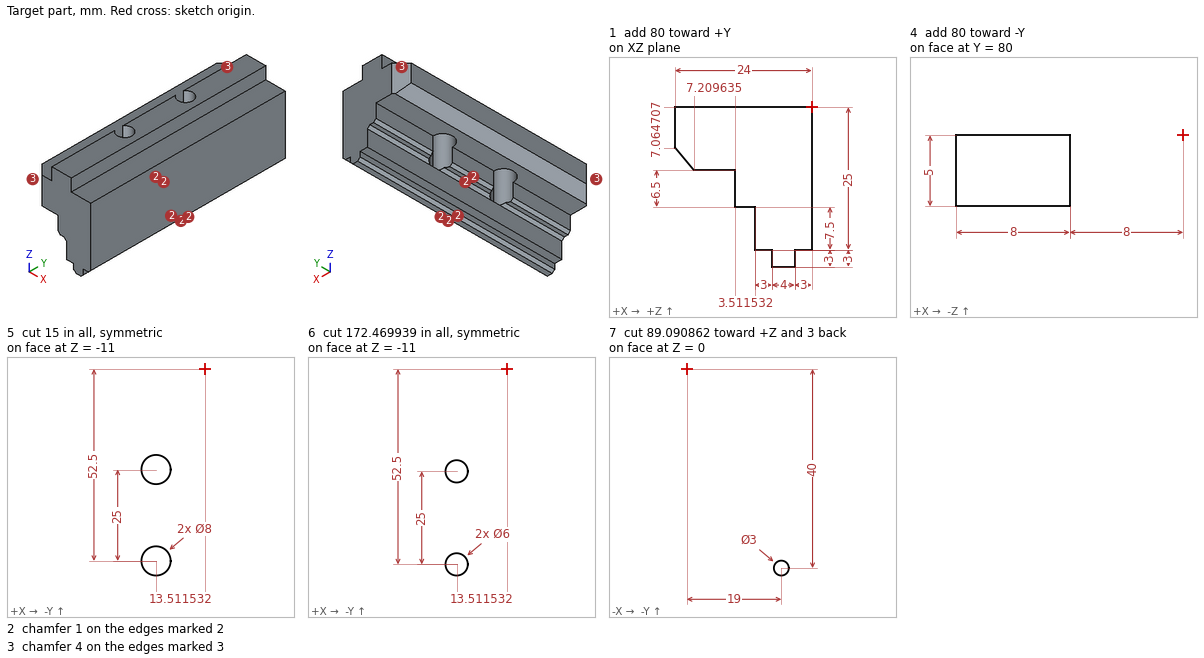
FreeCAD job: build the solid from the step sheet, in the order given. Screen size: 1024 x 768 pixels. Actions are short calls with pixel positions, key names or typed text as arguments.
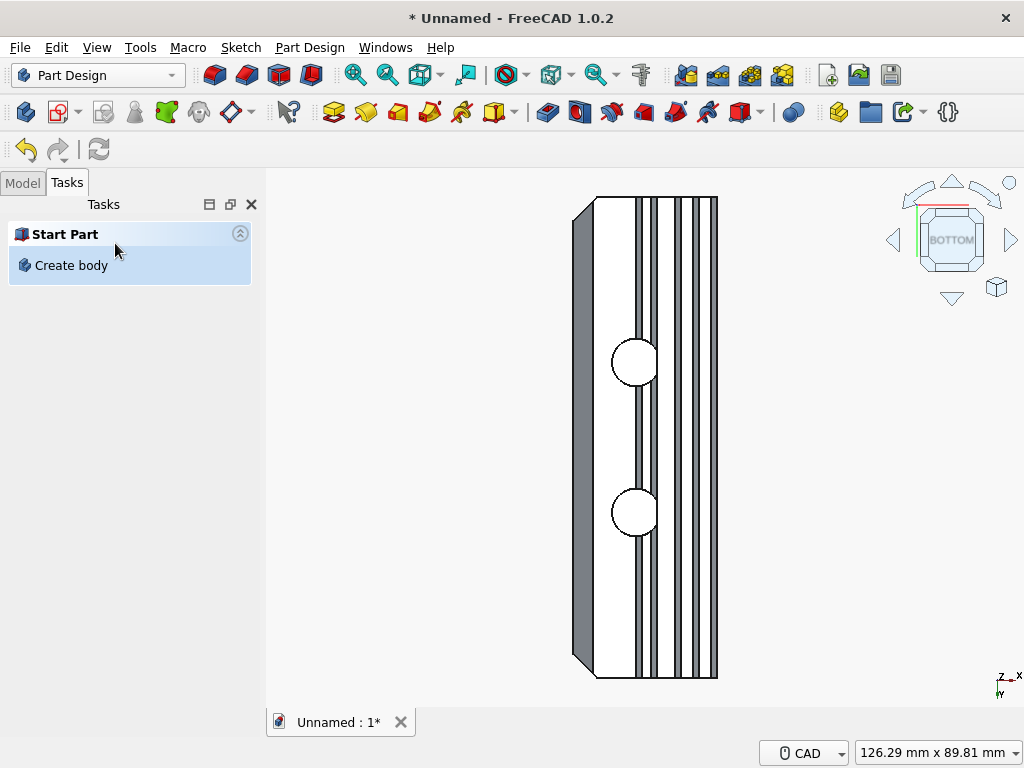
click(614, 642)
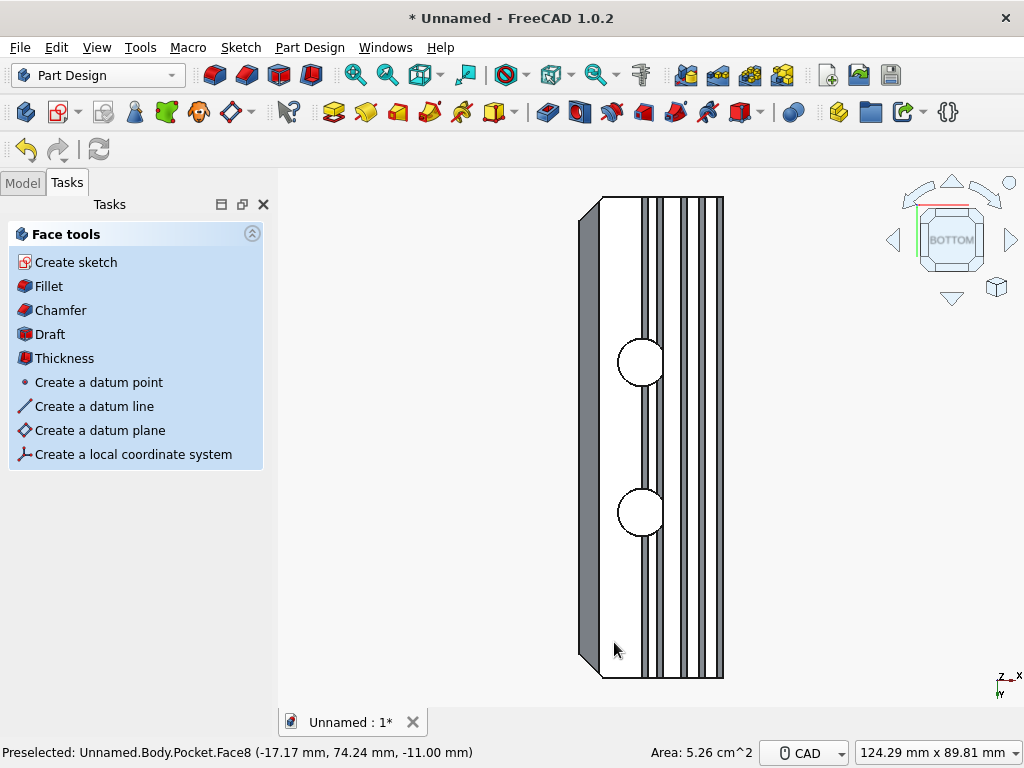
click(58, 112)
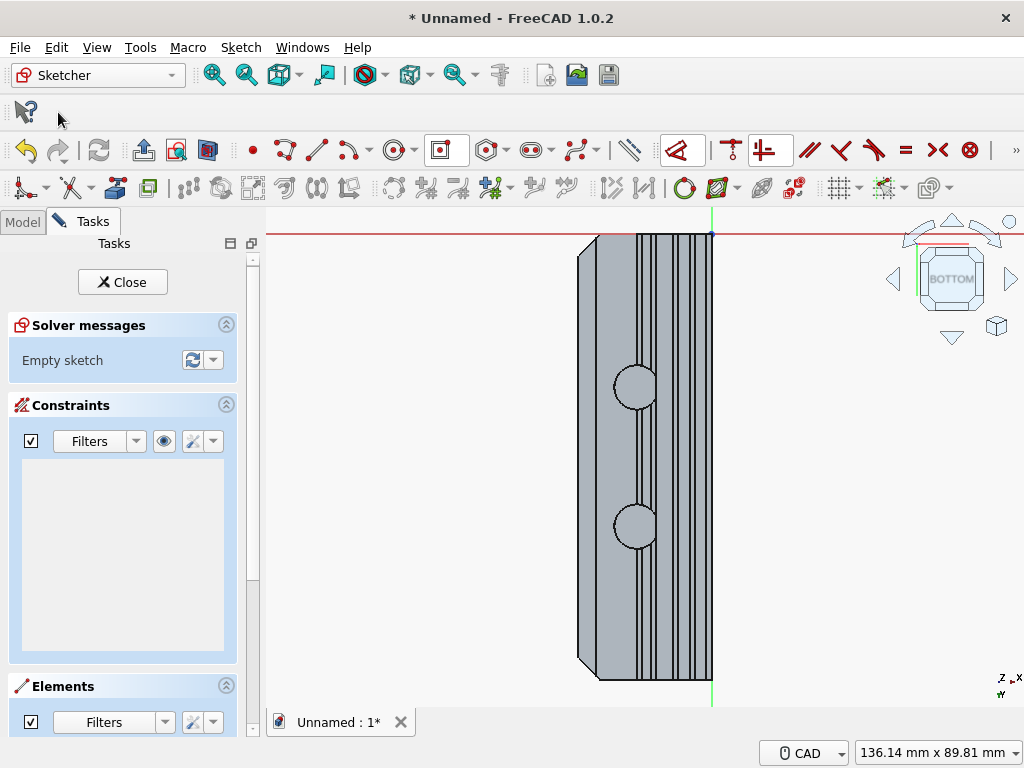
key(q)
key(s)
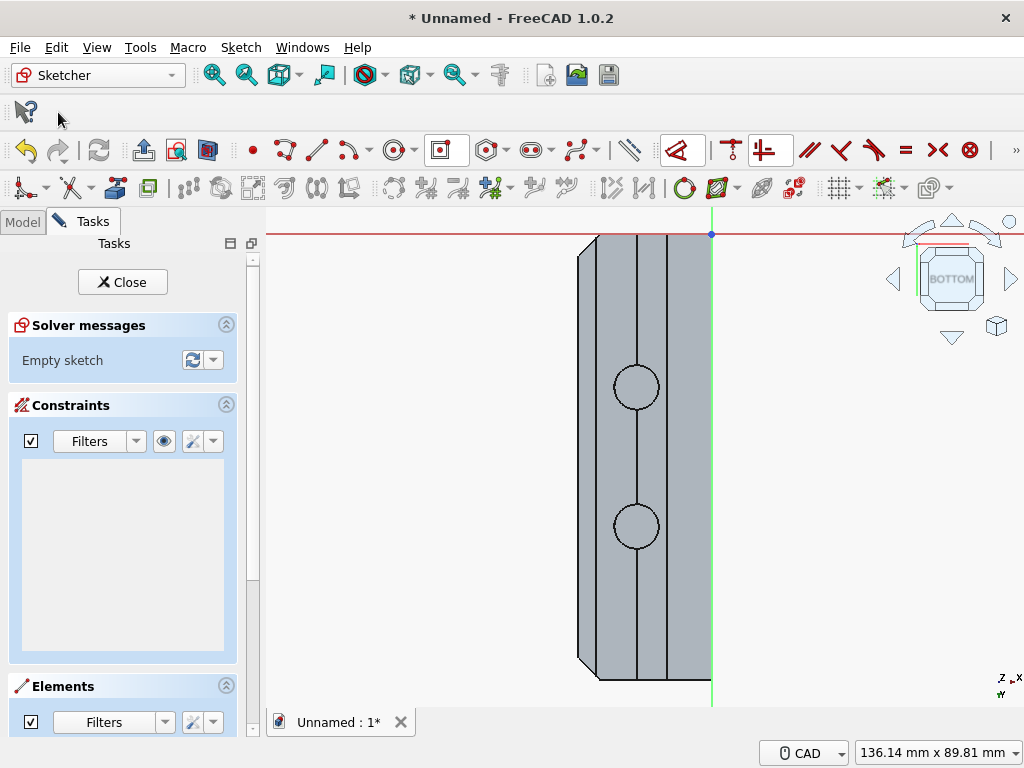
scroll(294, 679, down, 1)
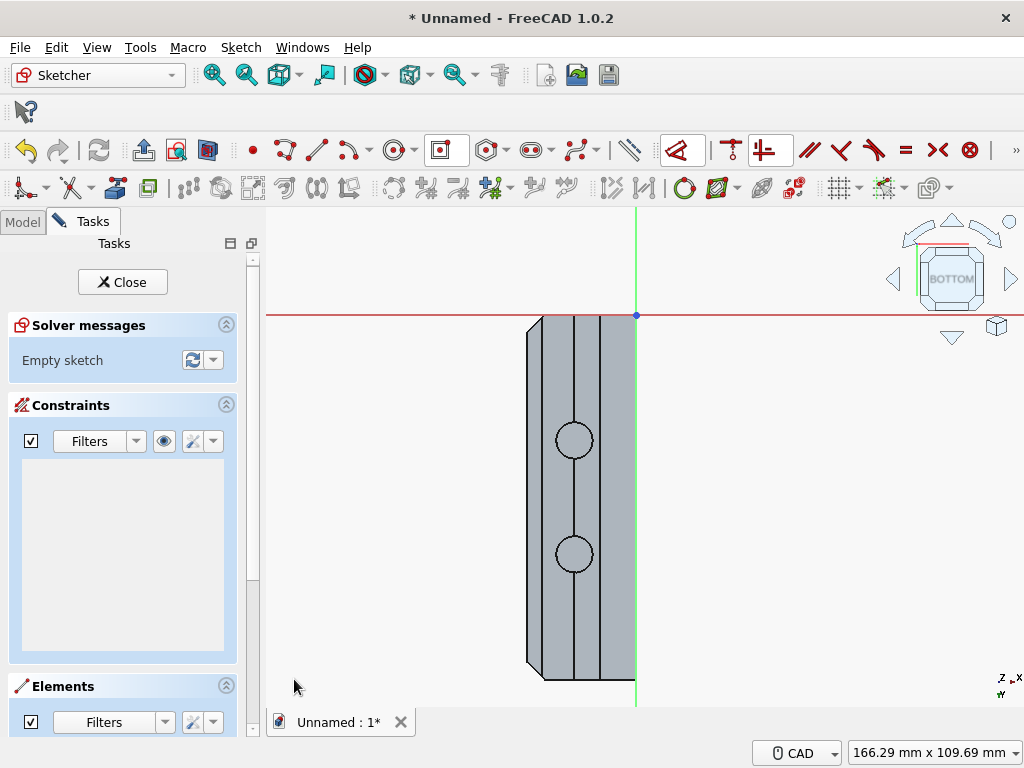
click(394, 150)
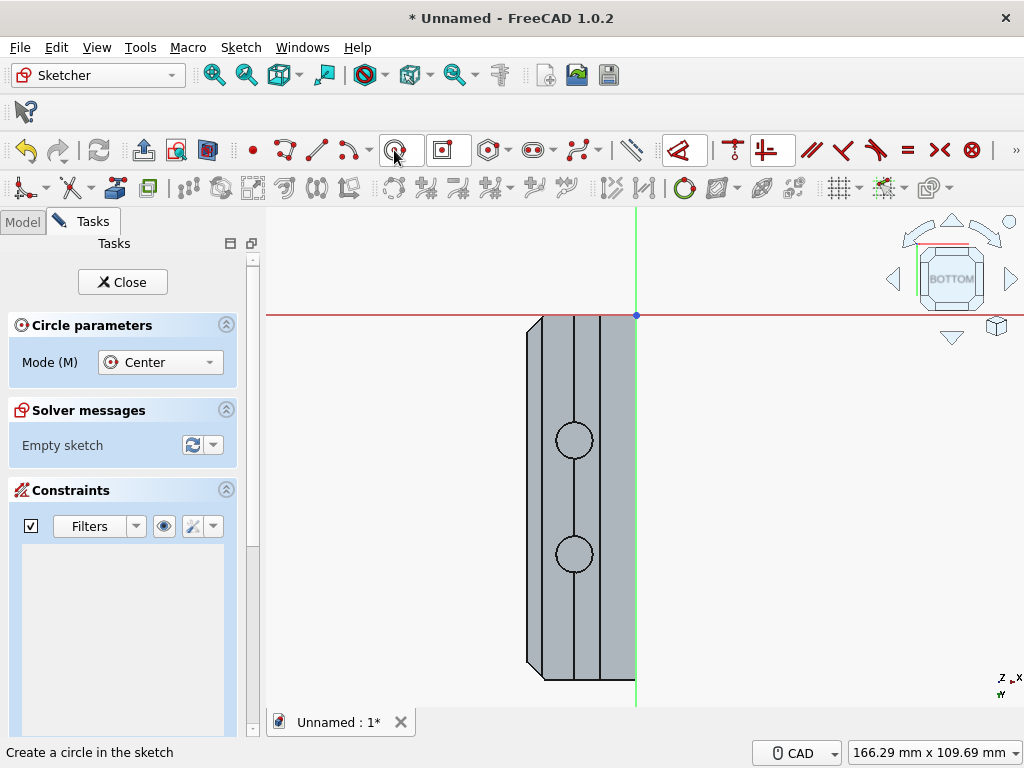
scroll(574, 554, up, 3)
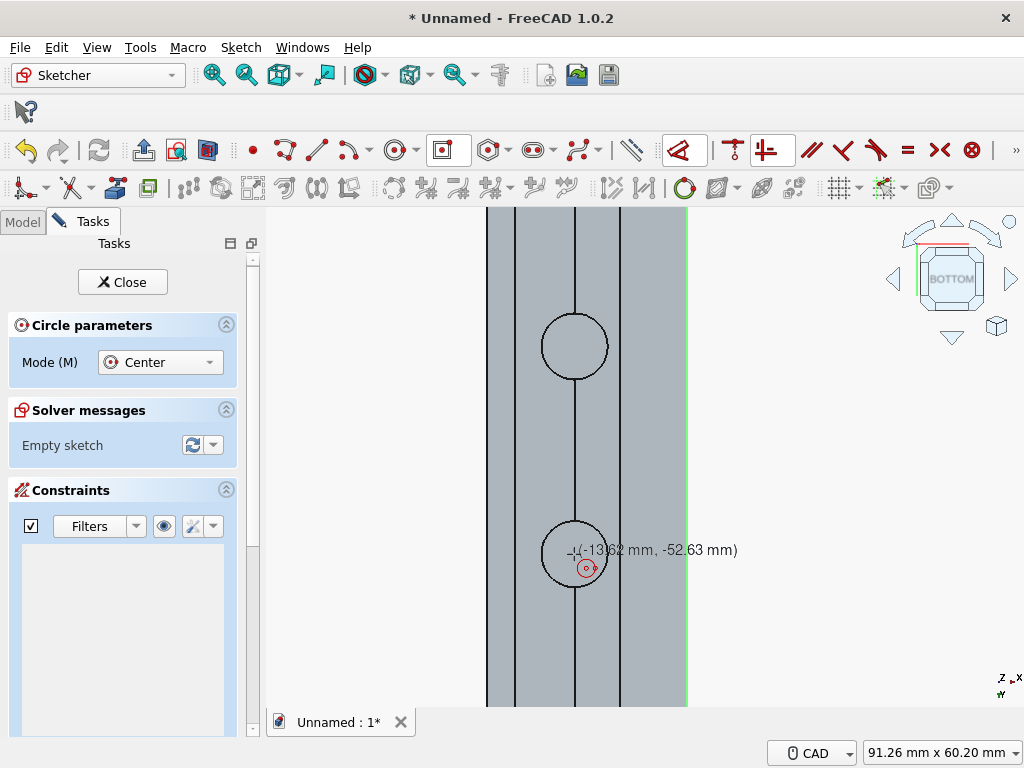
click(575, 554)
click(592, 537)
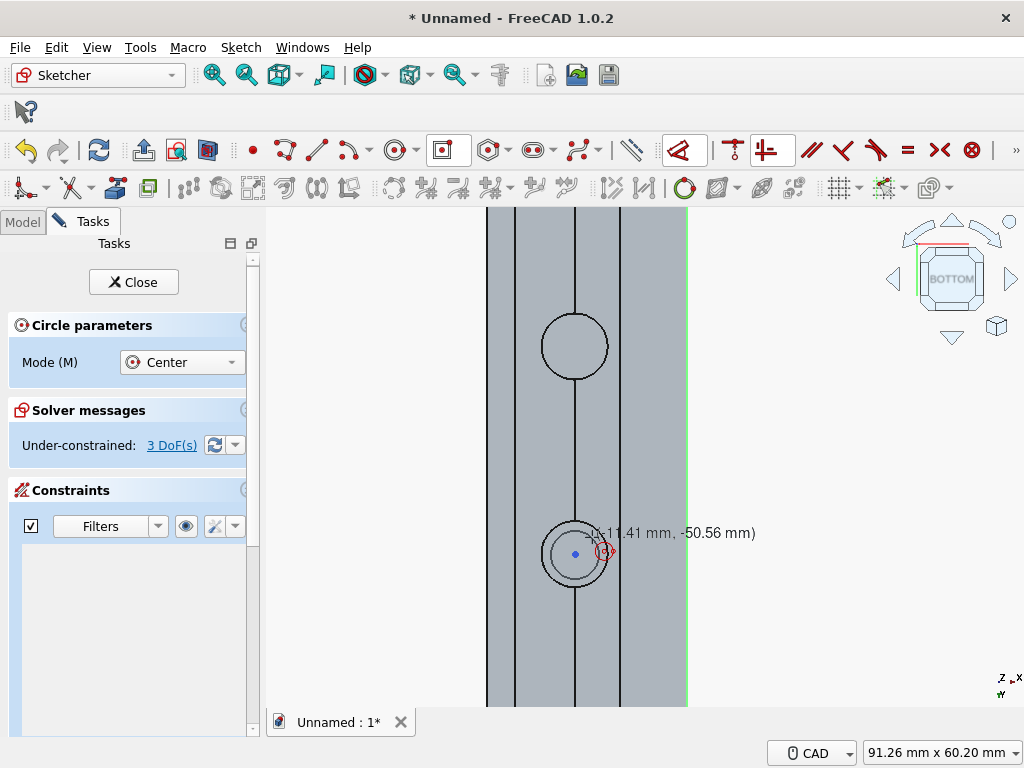
click(575, 346)
click(592, 329)
key(Escape)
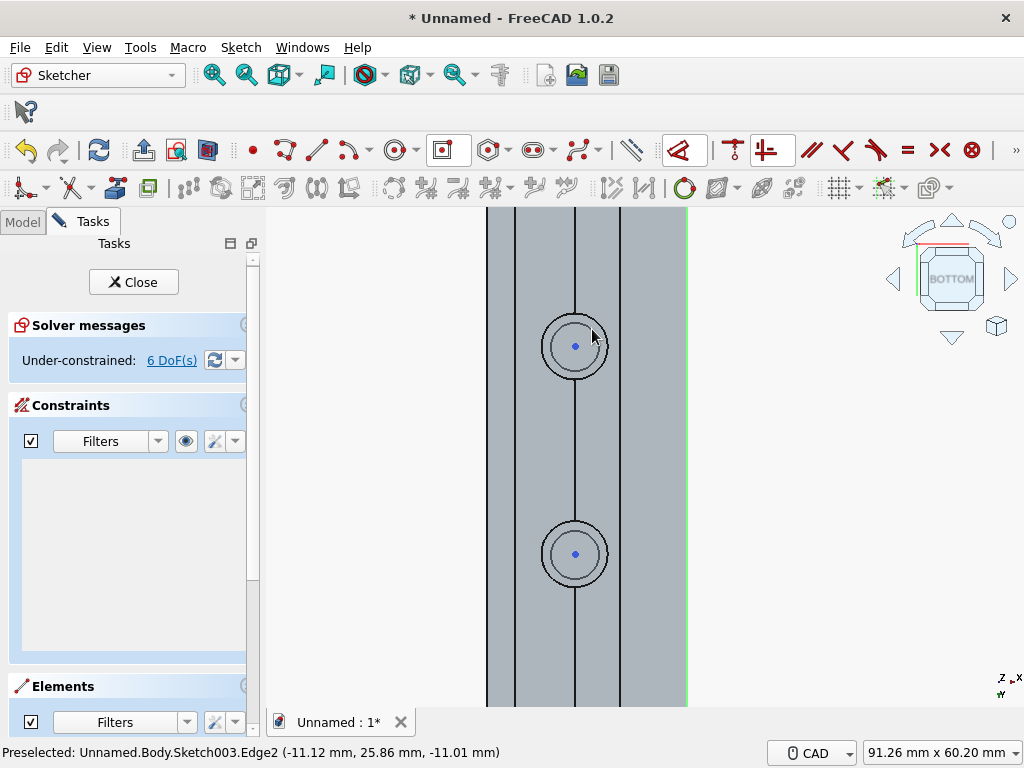
click(592, 538)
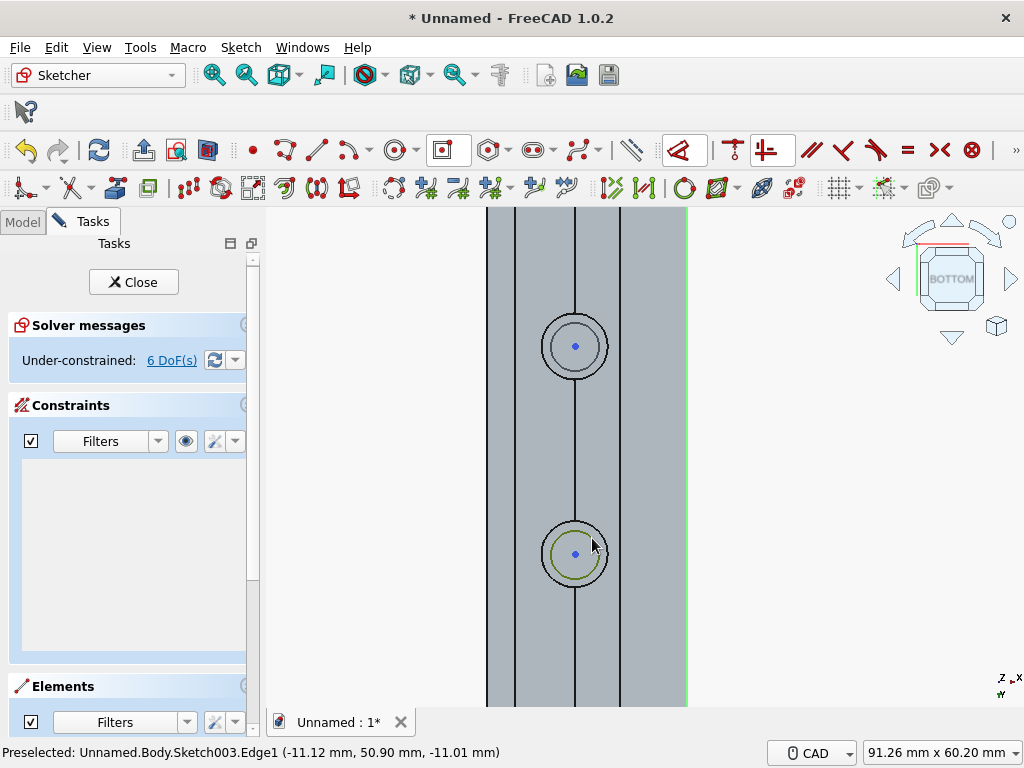
click(592, 330)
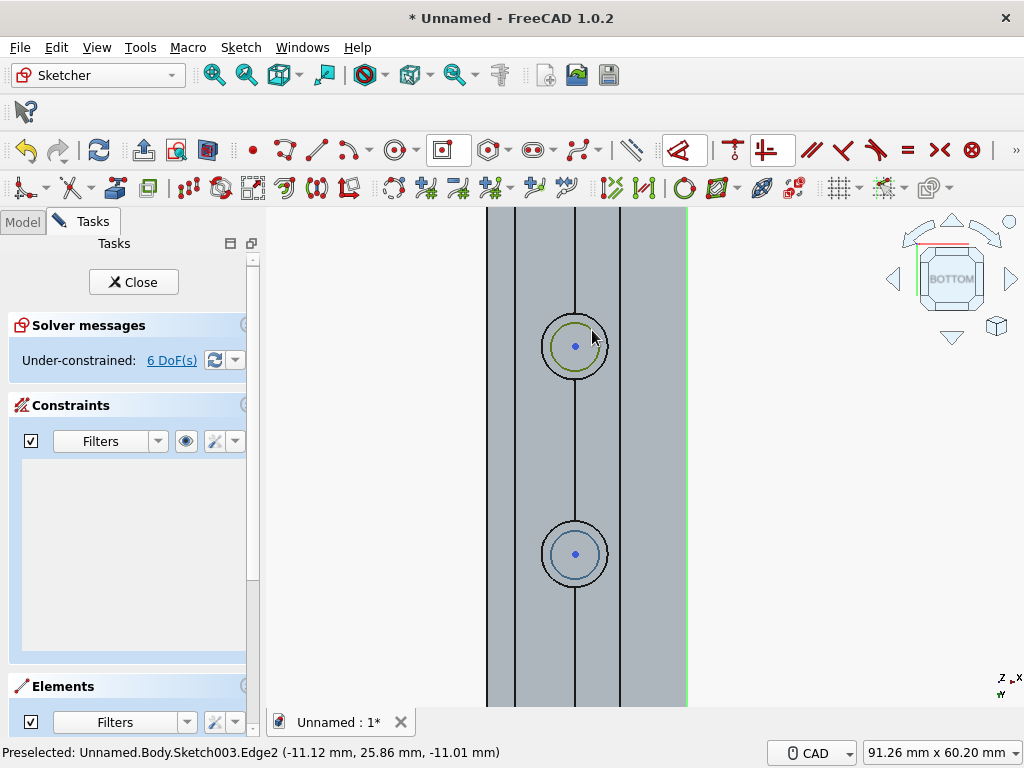
click(908, 150)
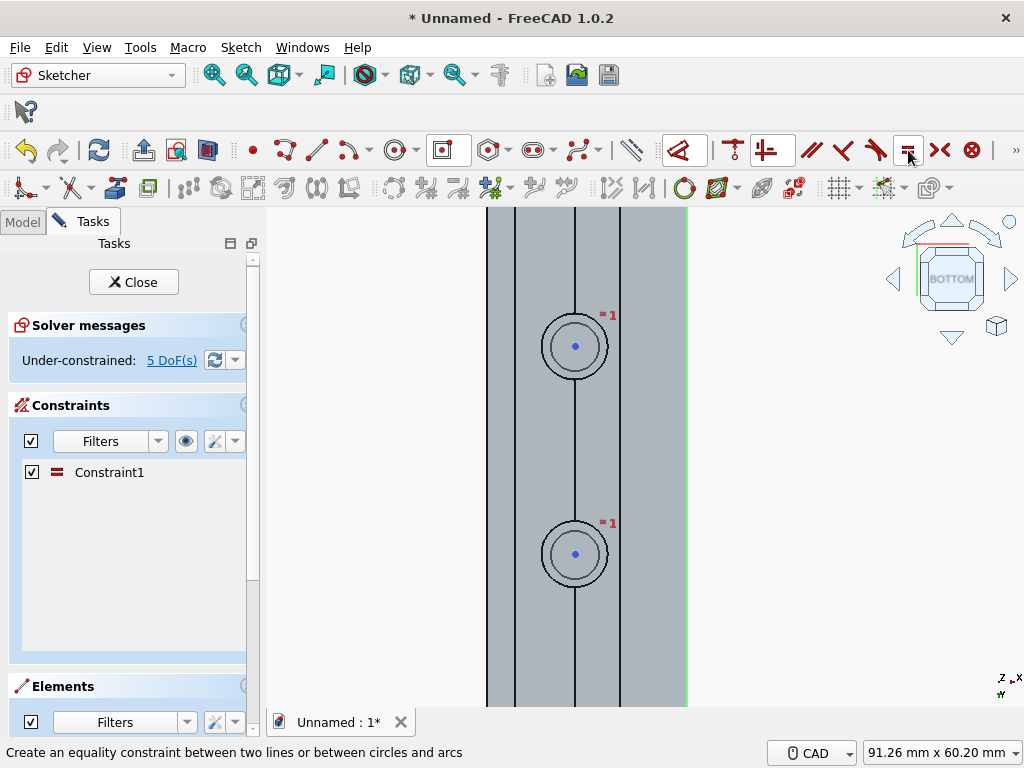
click(575, 555)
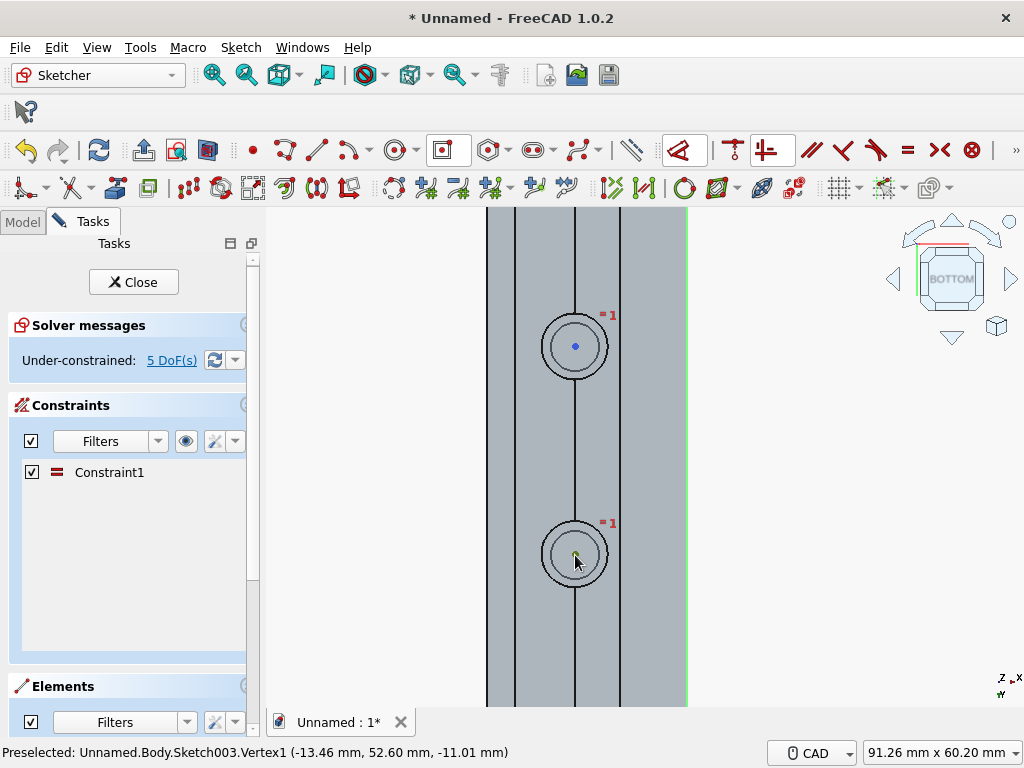
click(575, 347)